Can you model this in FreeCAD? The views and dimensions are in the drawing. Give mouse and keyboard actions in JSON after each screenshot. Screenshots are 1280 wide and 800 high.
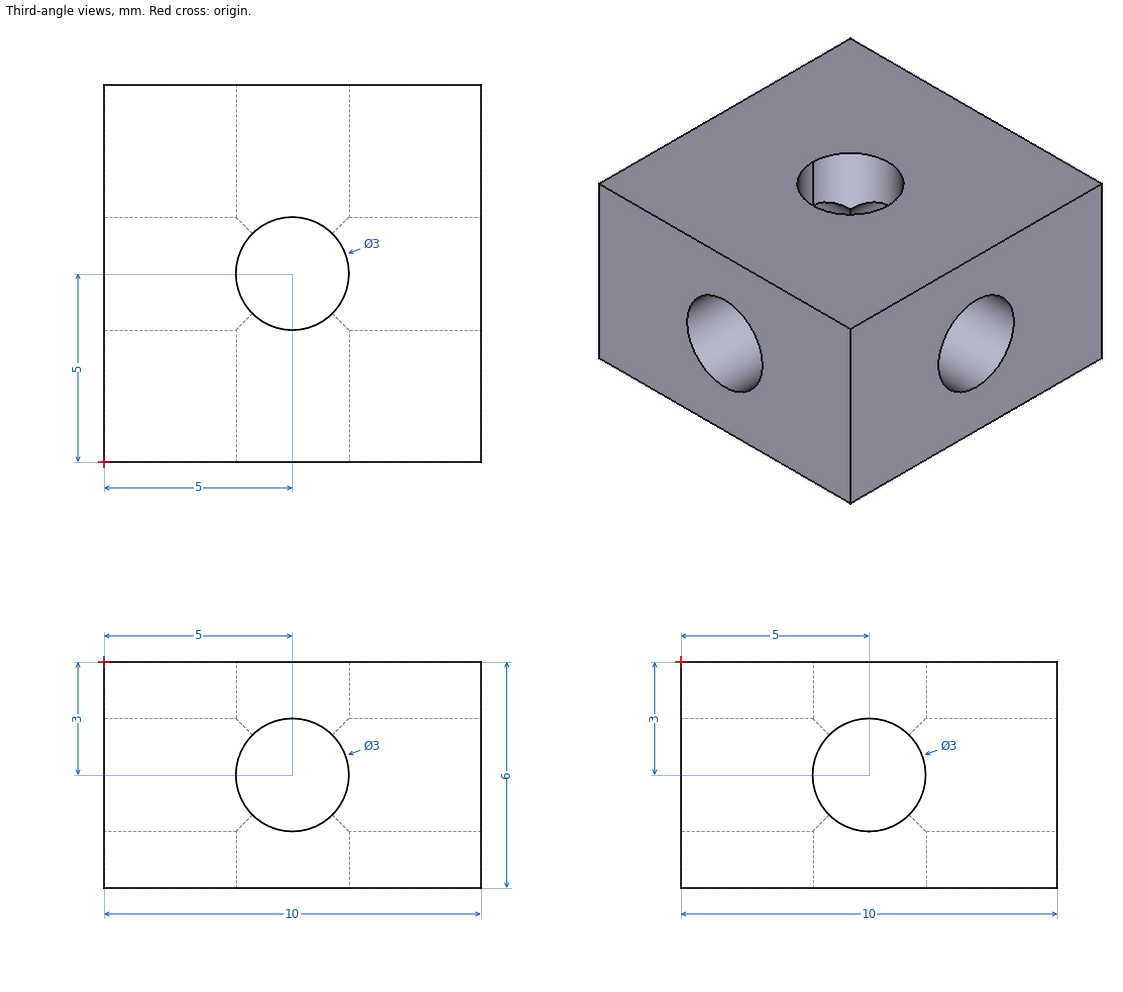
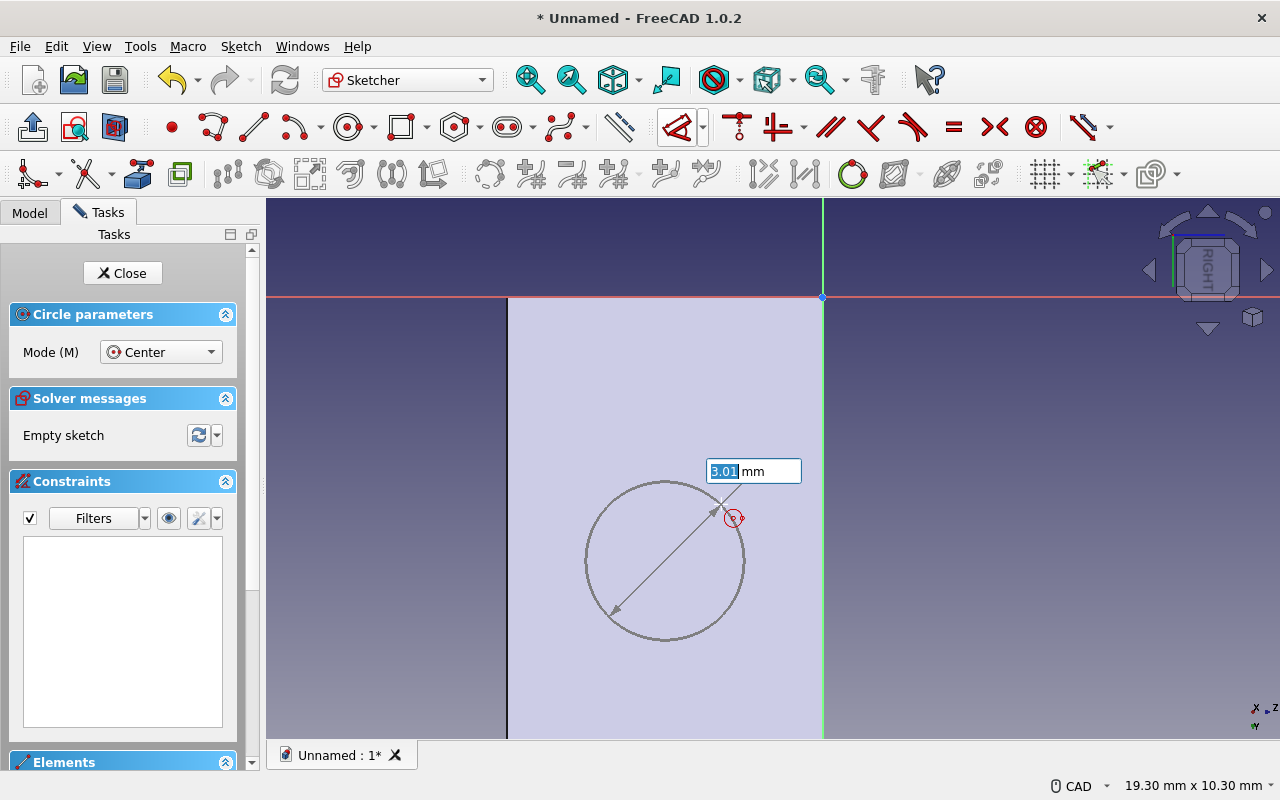
{"action": "type", "text": "3"}
{"action": "key", "text": "Return"}
{"action": "key", "text": "Escape"}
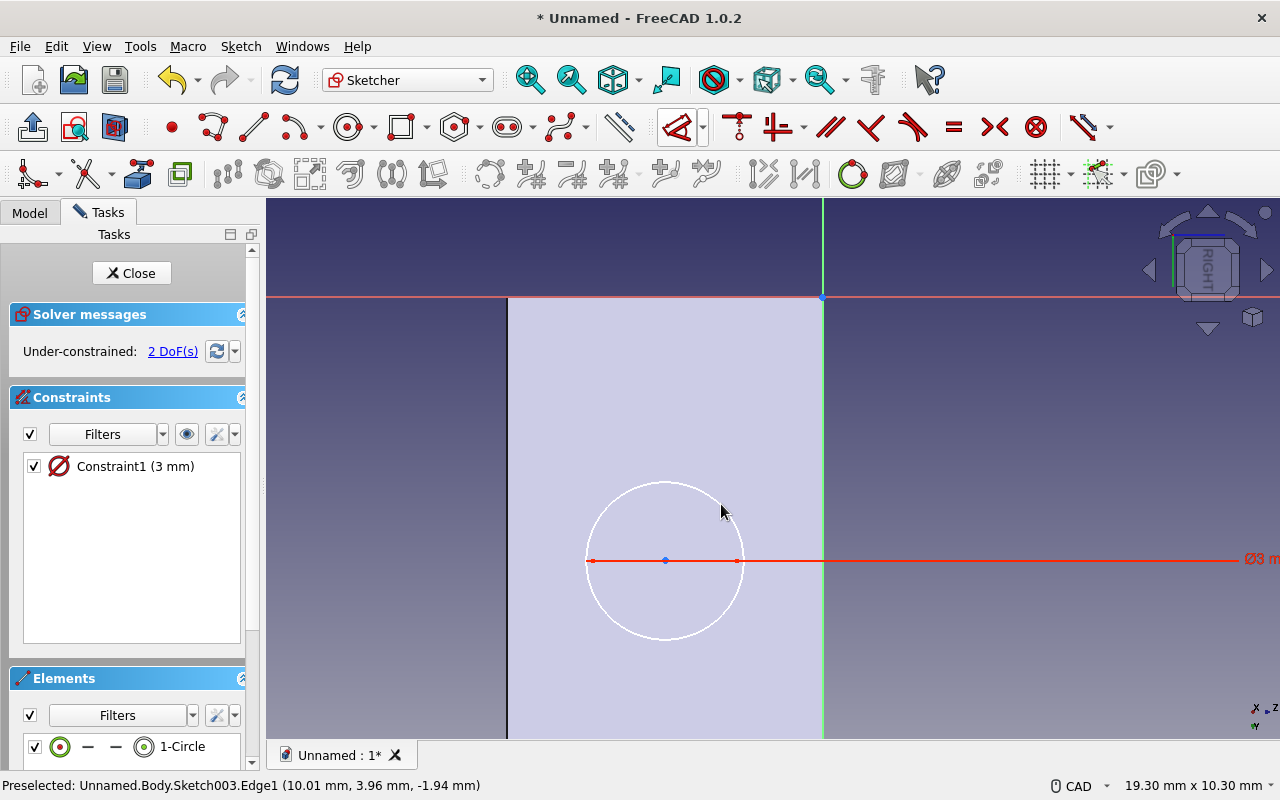
{"action": "left_click", "coordinate": [665, 561]}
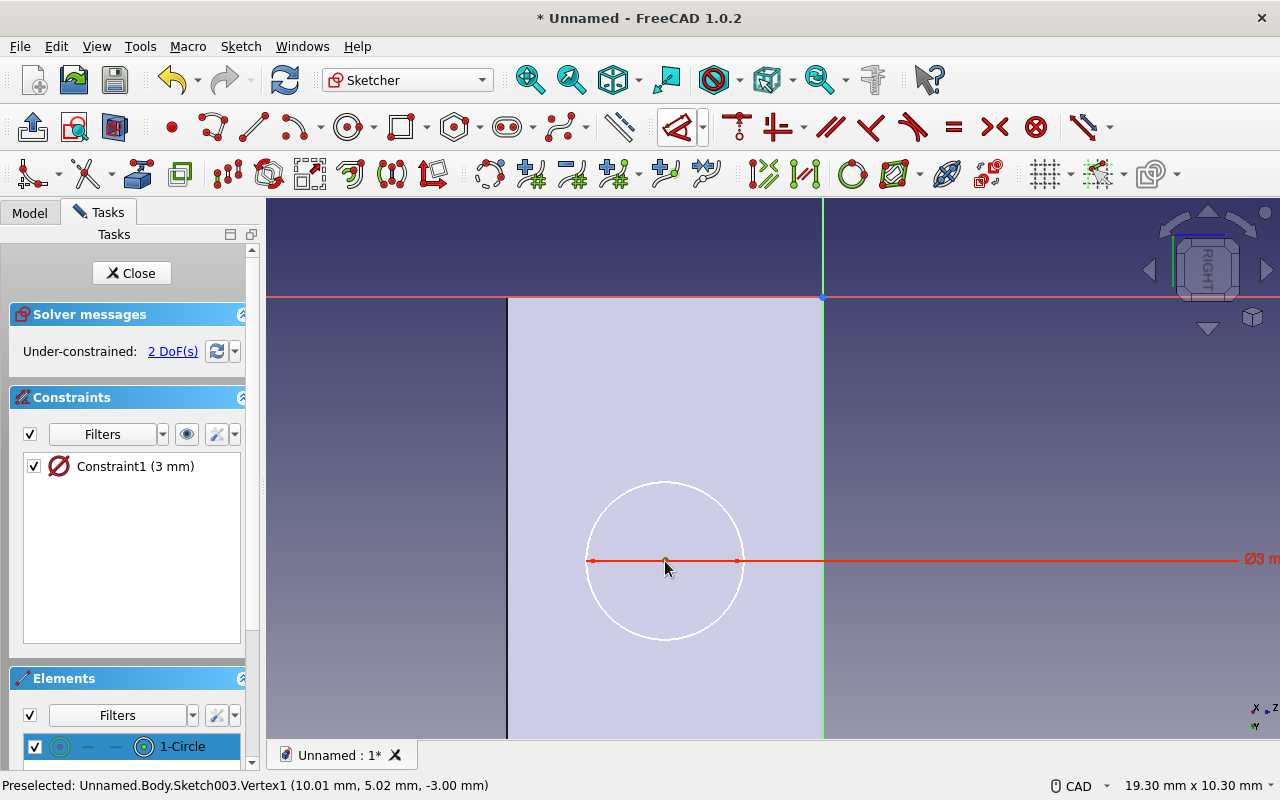
{"action": "key", "text": "l"}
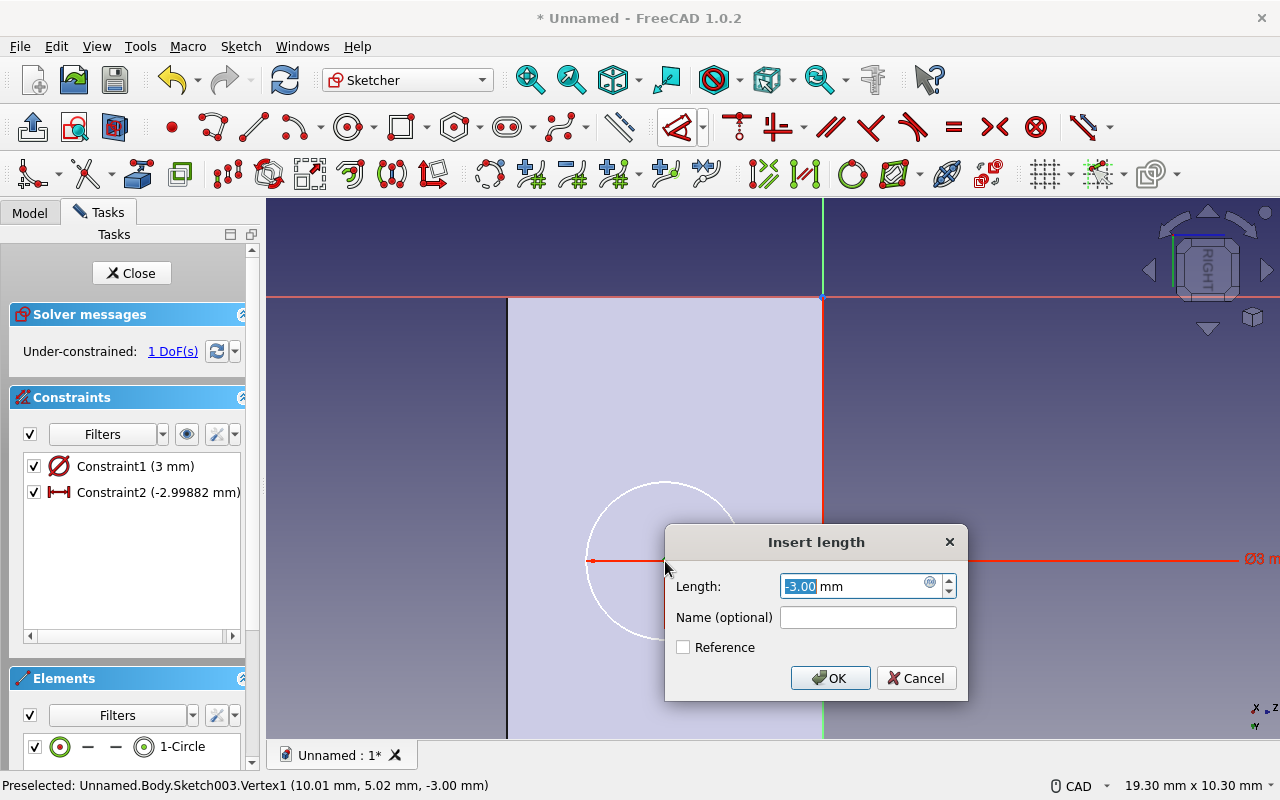
{"action": "type", "text": "-3"}
{"action": "key", "text": "Return"}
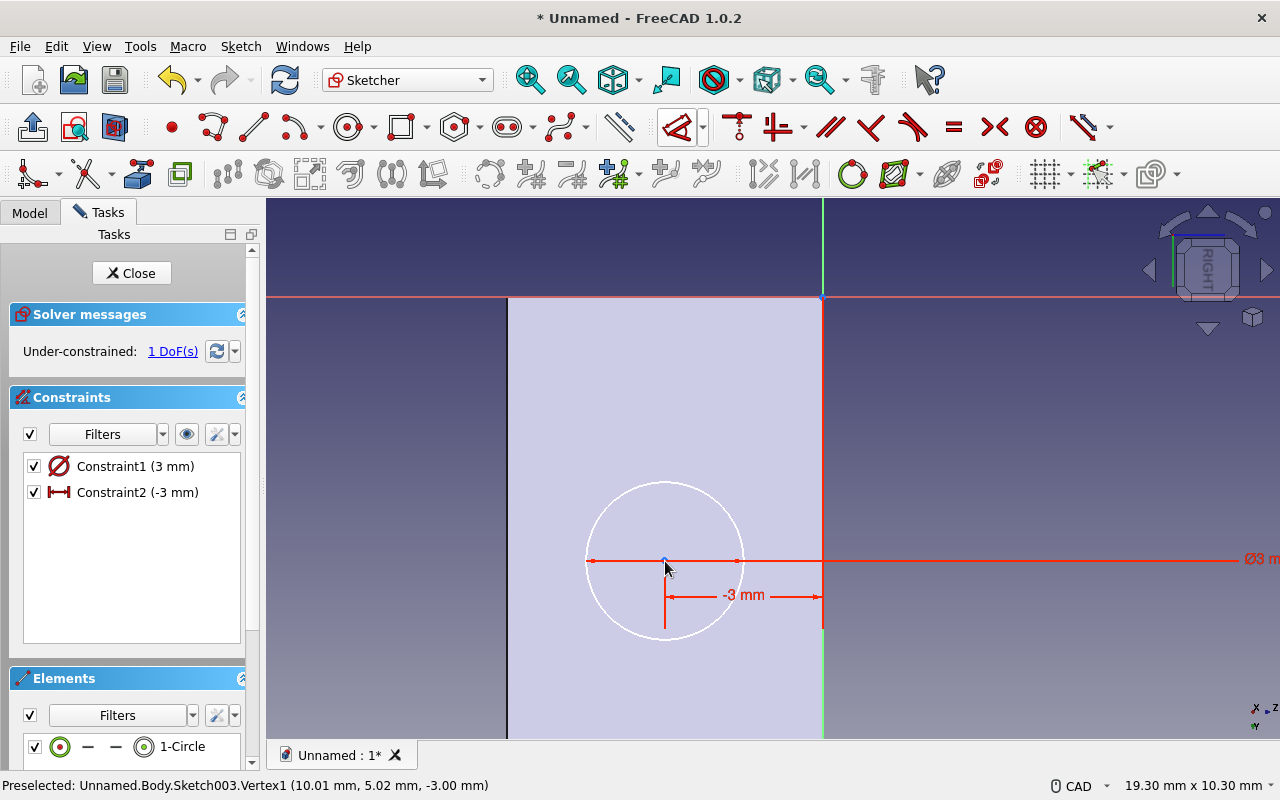
{"action": "left_click", "coordinate": [665, 561]}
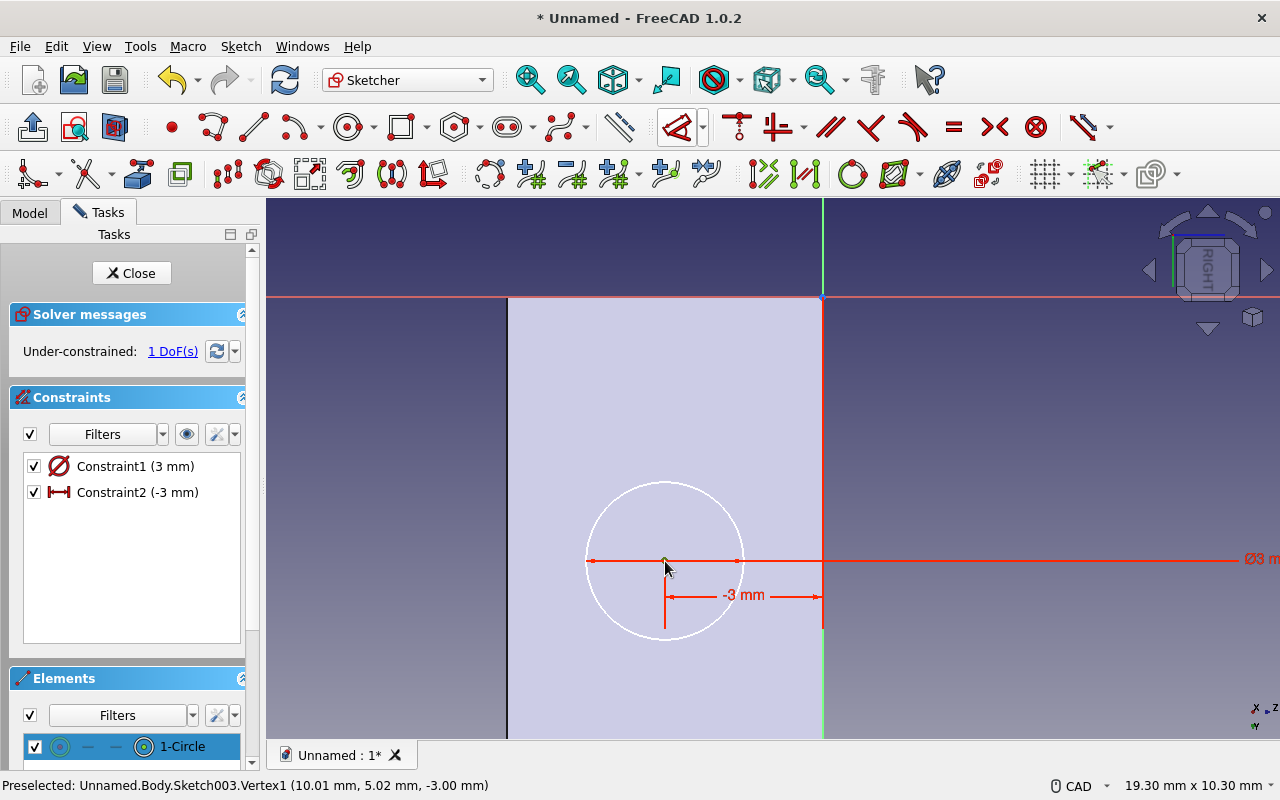
{"action": "left_click", "coordinate": [702, 128]}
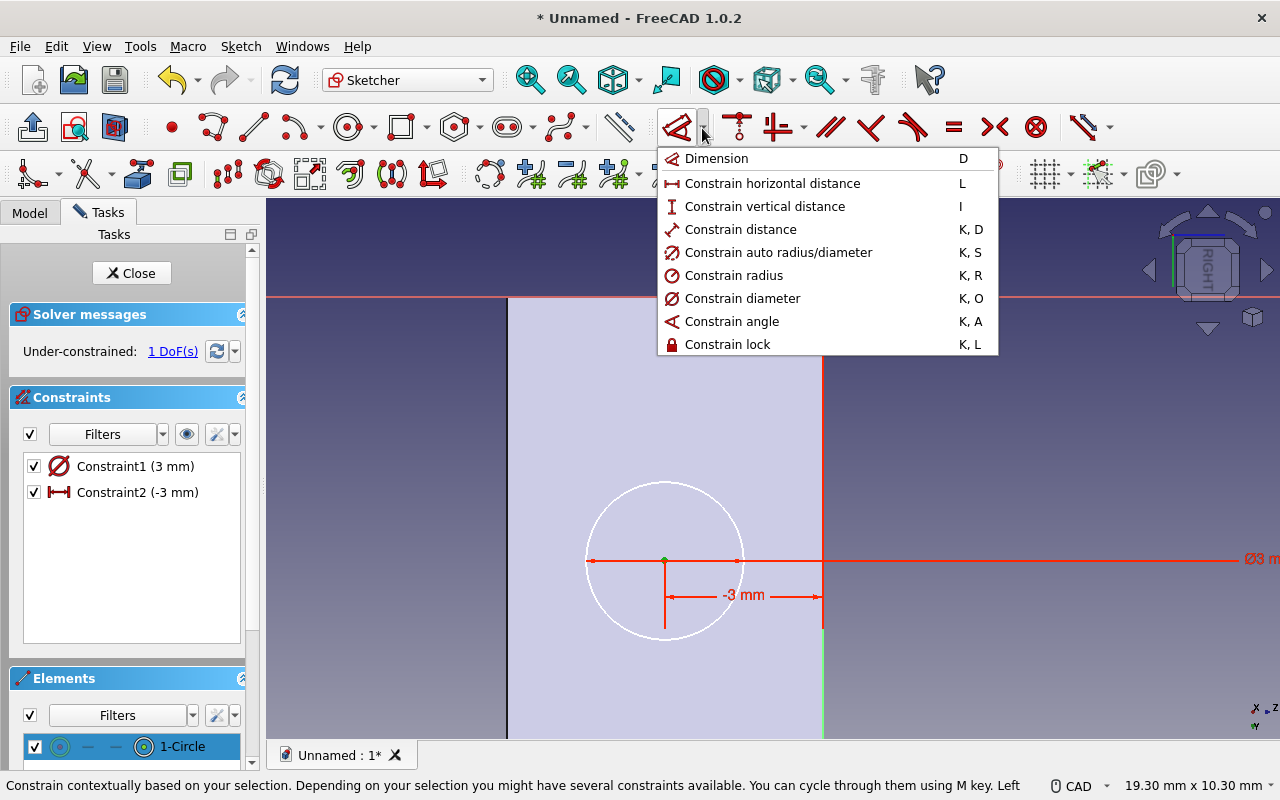
{"action": "left_click", "coordinate": [828, 206]}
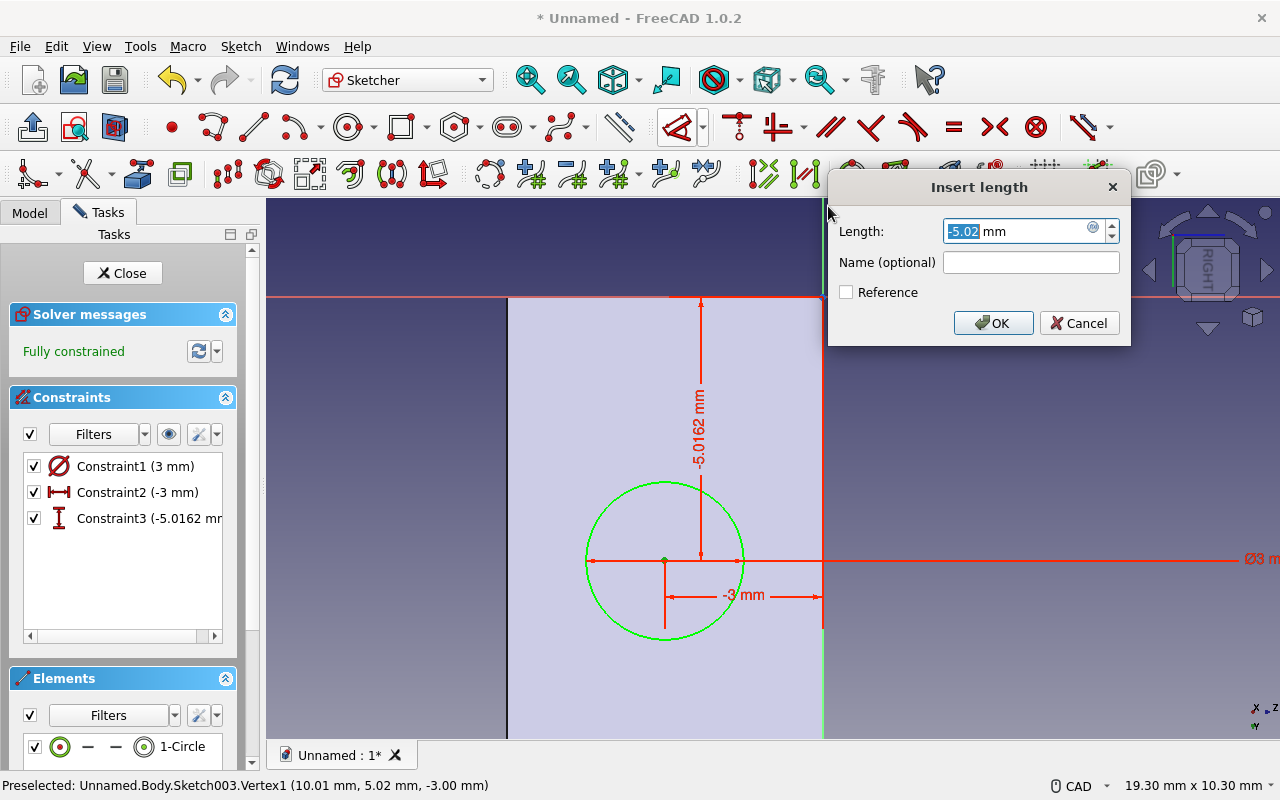
{"action": "type", "text": "-5"}
{"action": "key", "text": "Return"}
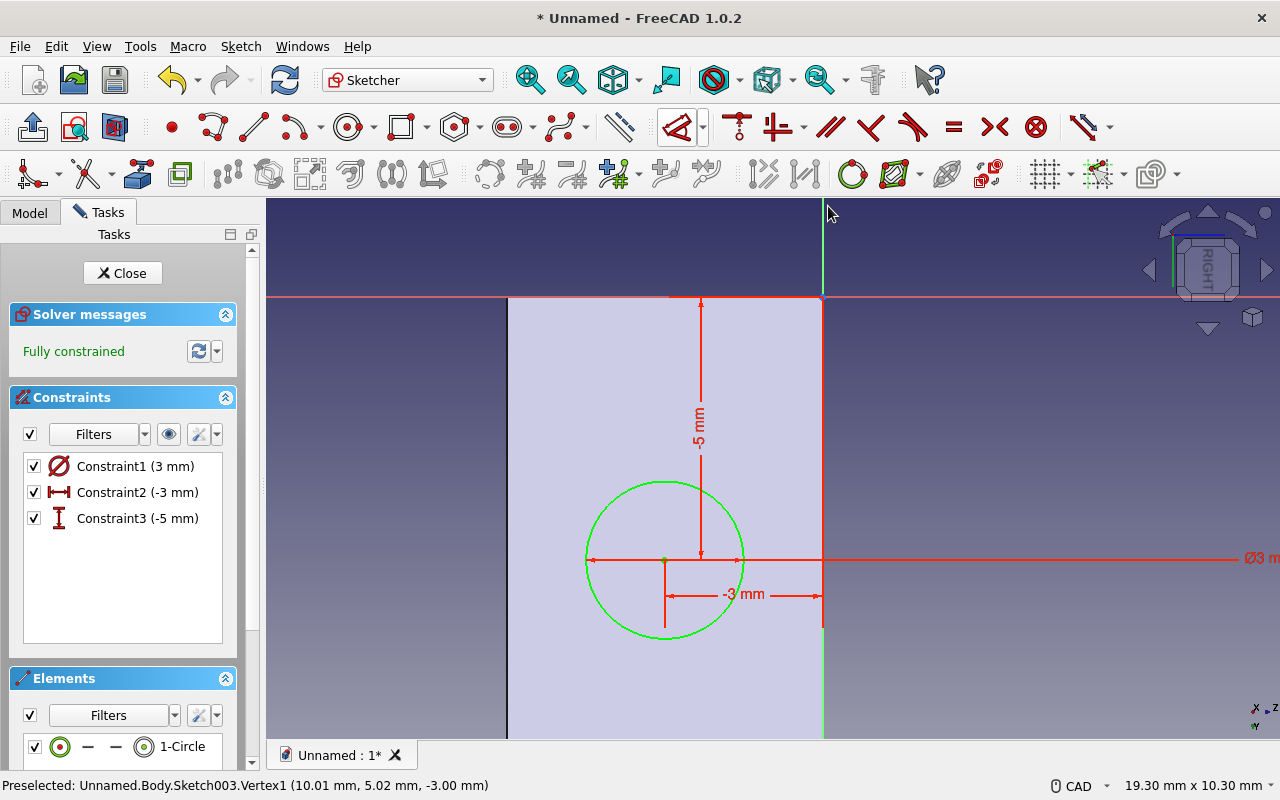
{"action": "left_click", "coordinate": [123, 273]}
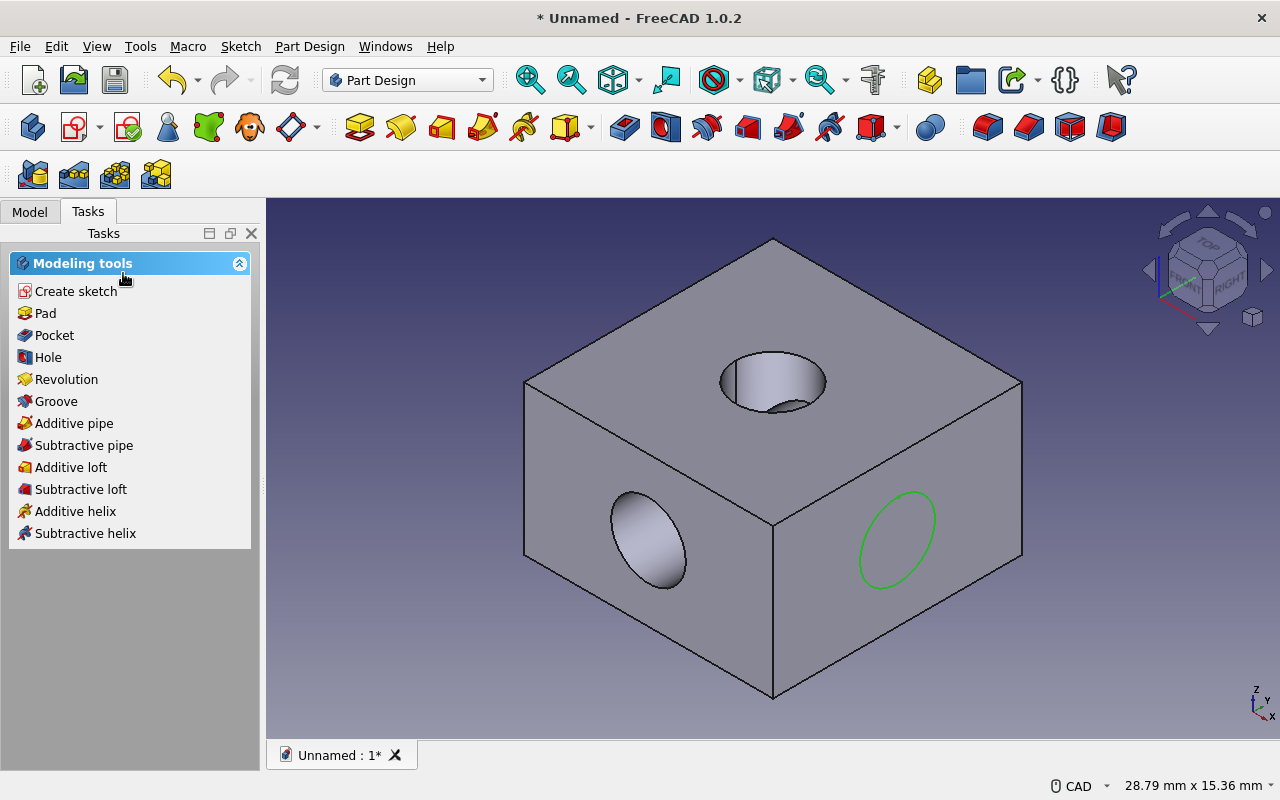
{"action": "left_click", "coordinate": [625, 128]}